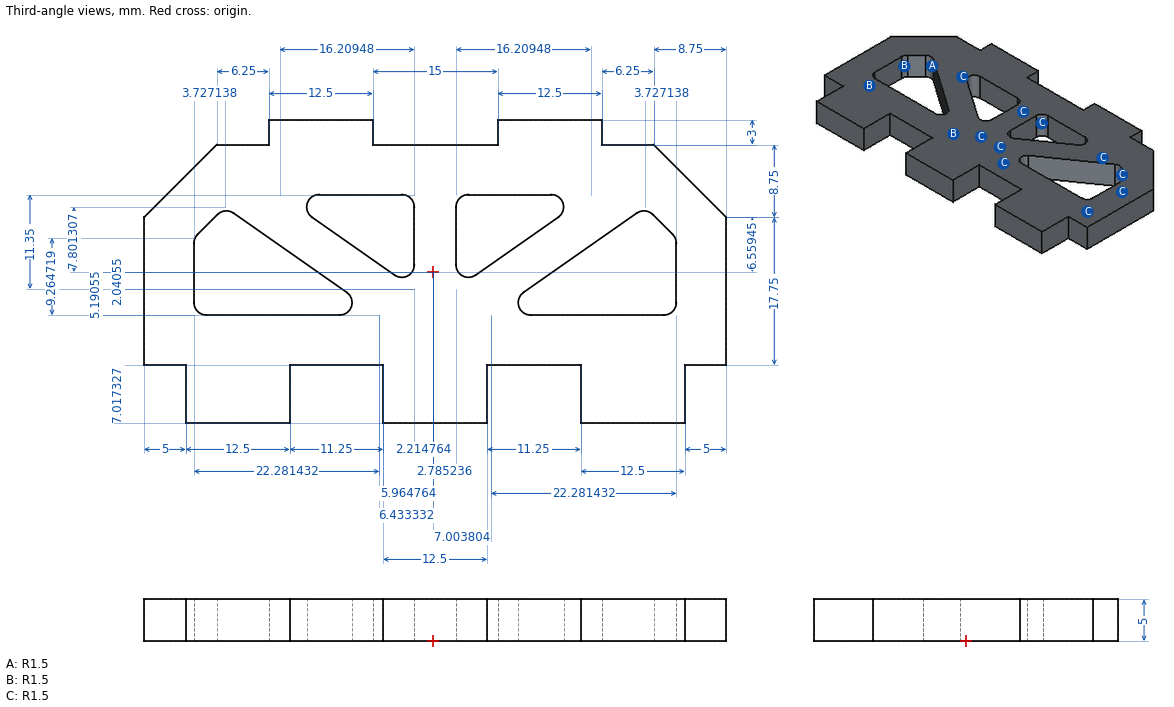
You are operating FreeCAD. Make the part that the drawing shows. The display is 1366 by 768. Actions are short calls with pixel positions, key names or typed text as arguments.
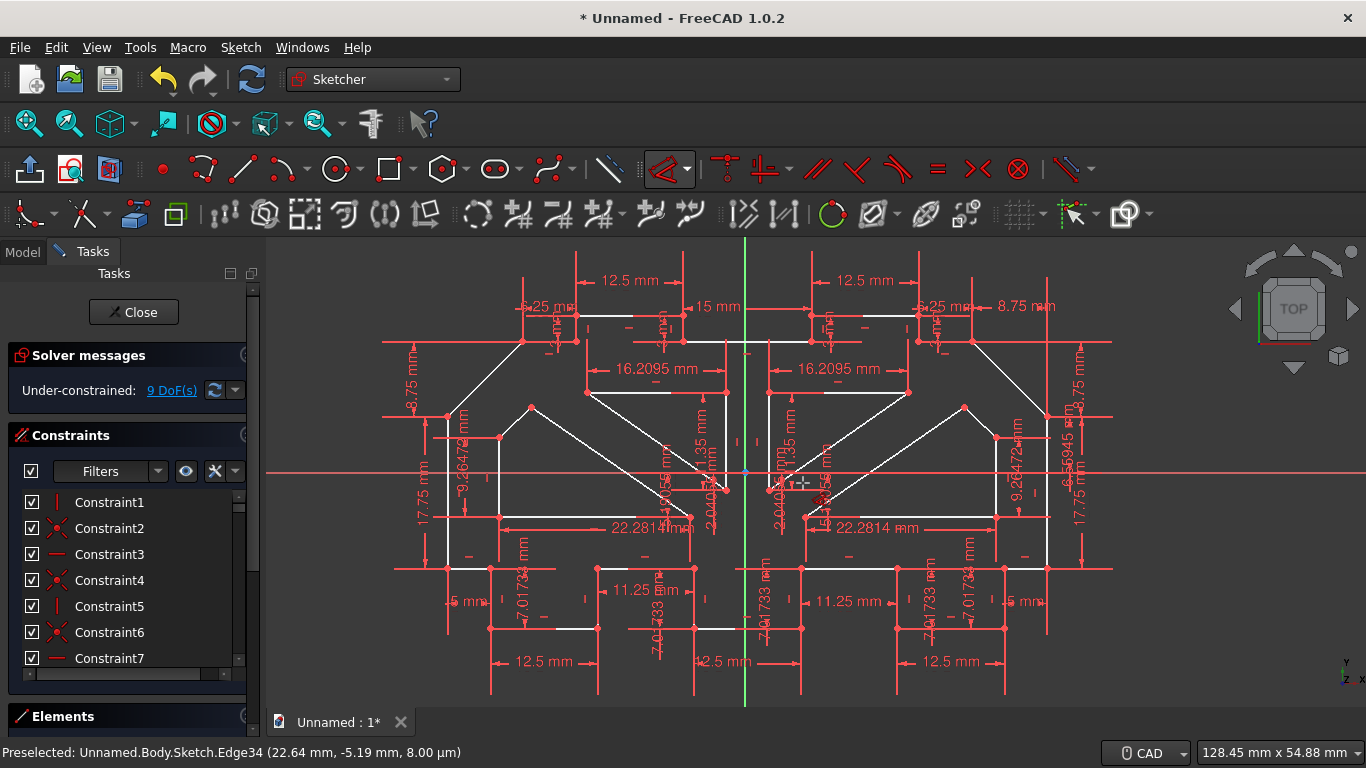
click(694, 569)
click(708, 415)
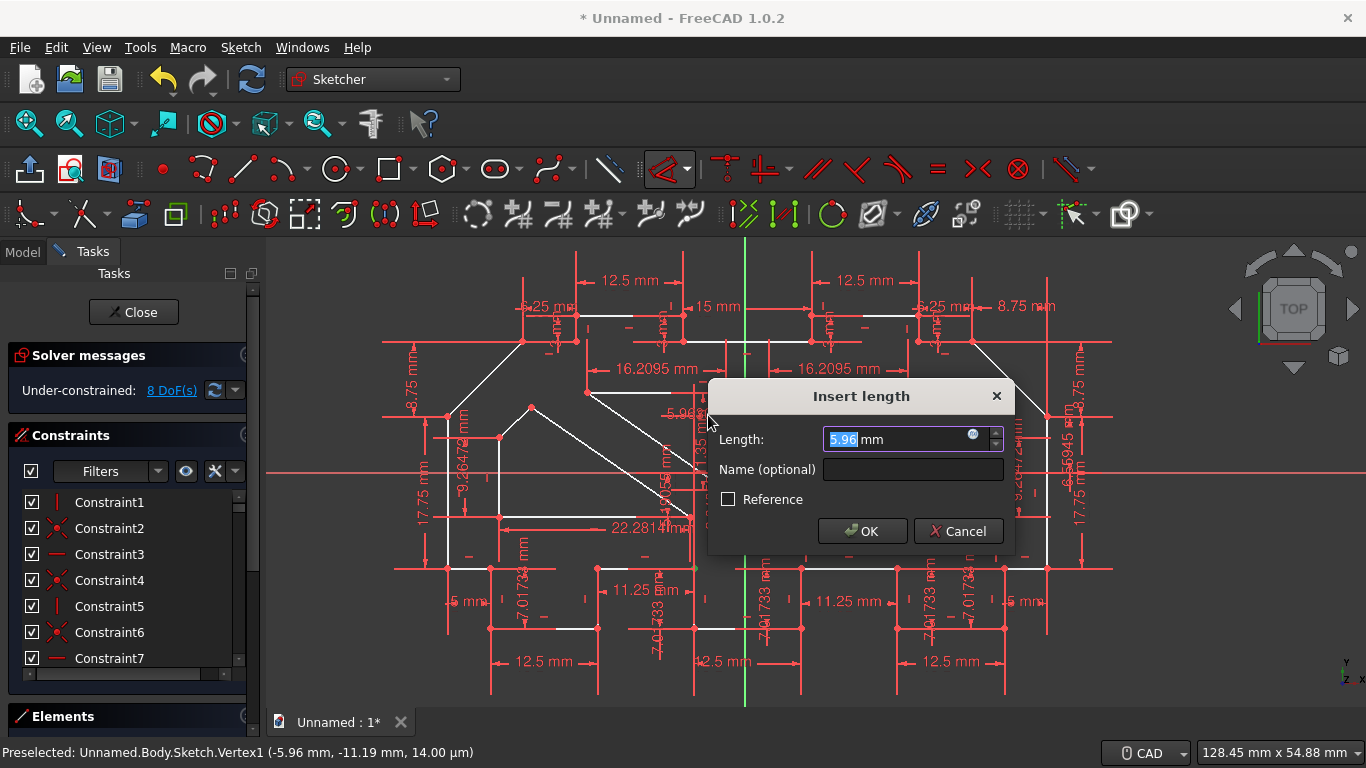
text(5.964764)
key(Return)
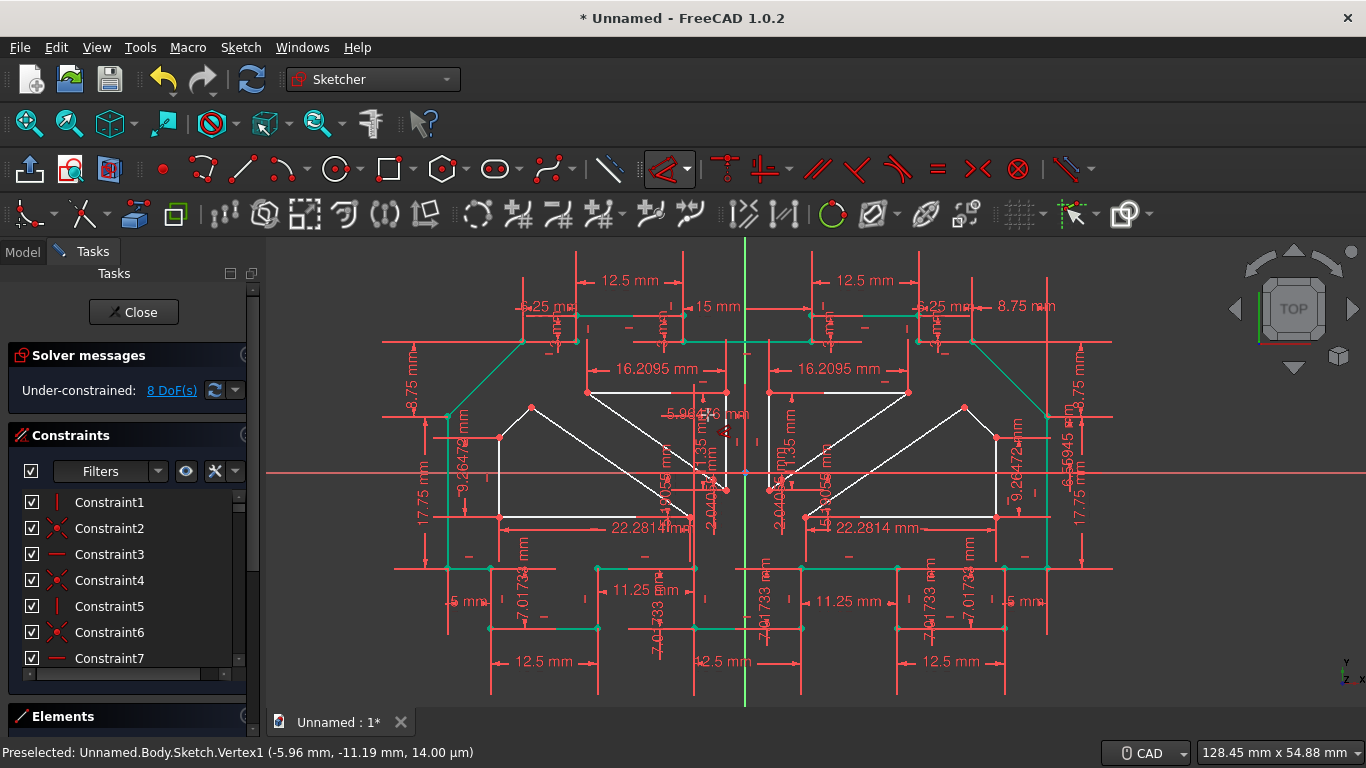
click(690, 517)
click(718, 551)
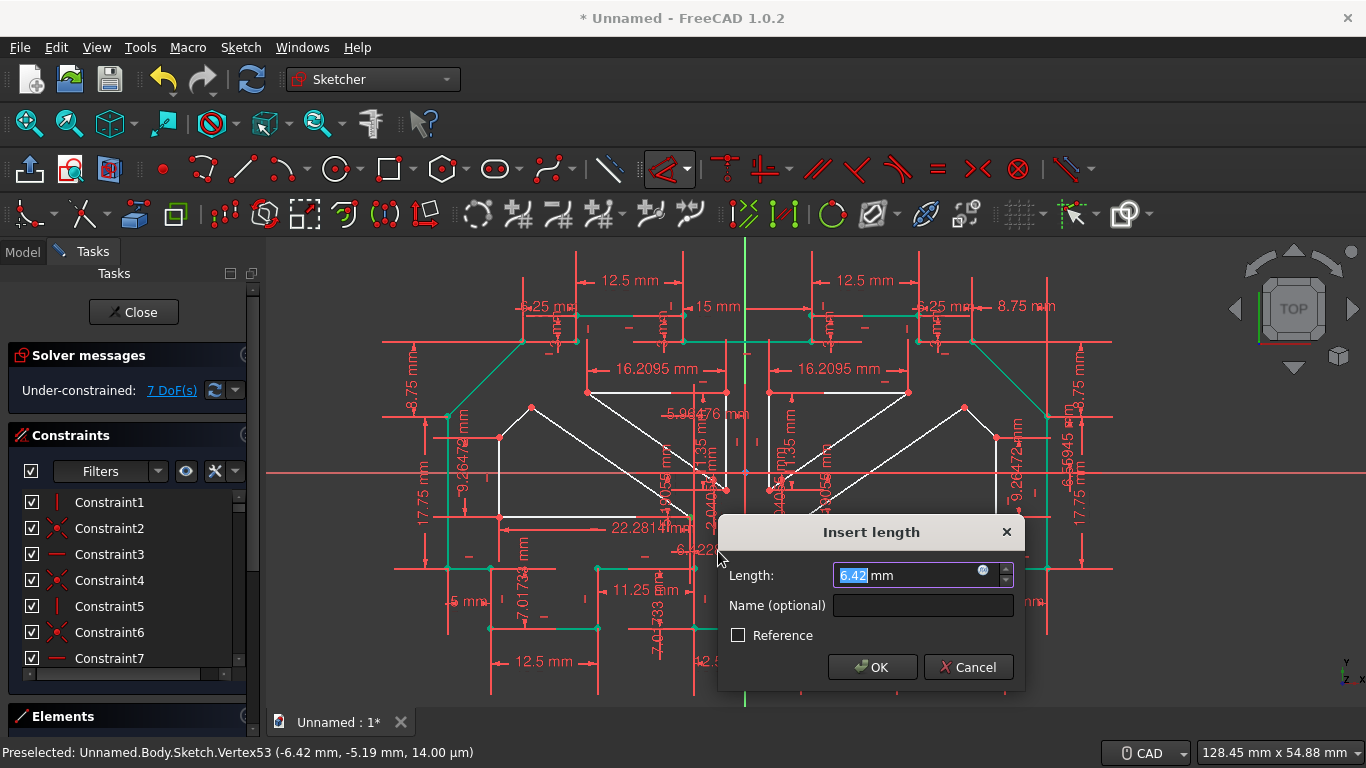
text(6.433332)
key(Return)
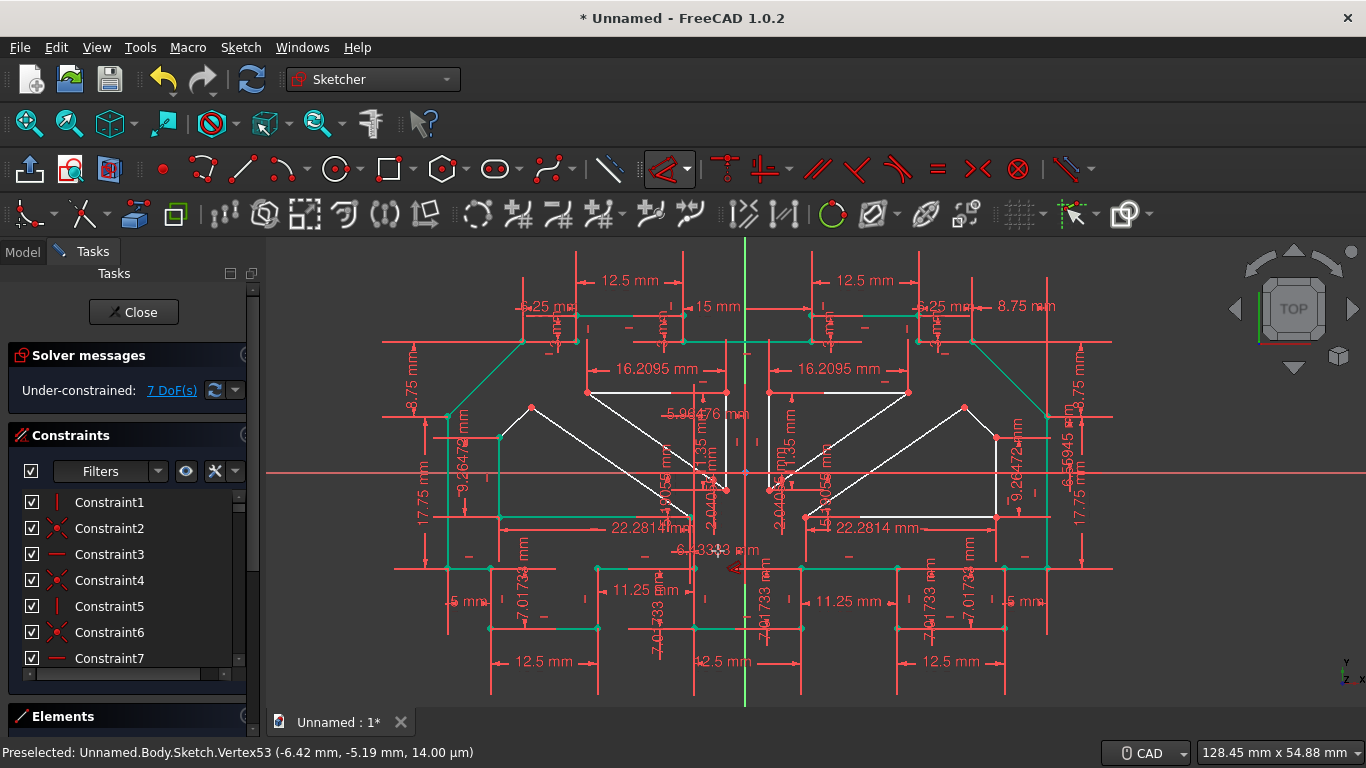
click(531, 407)
click(497, 417)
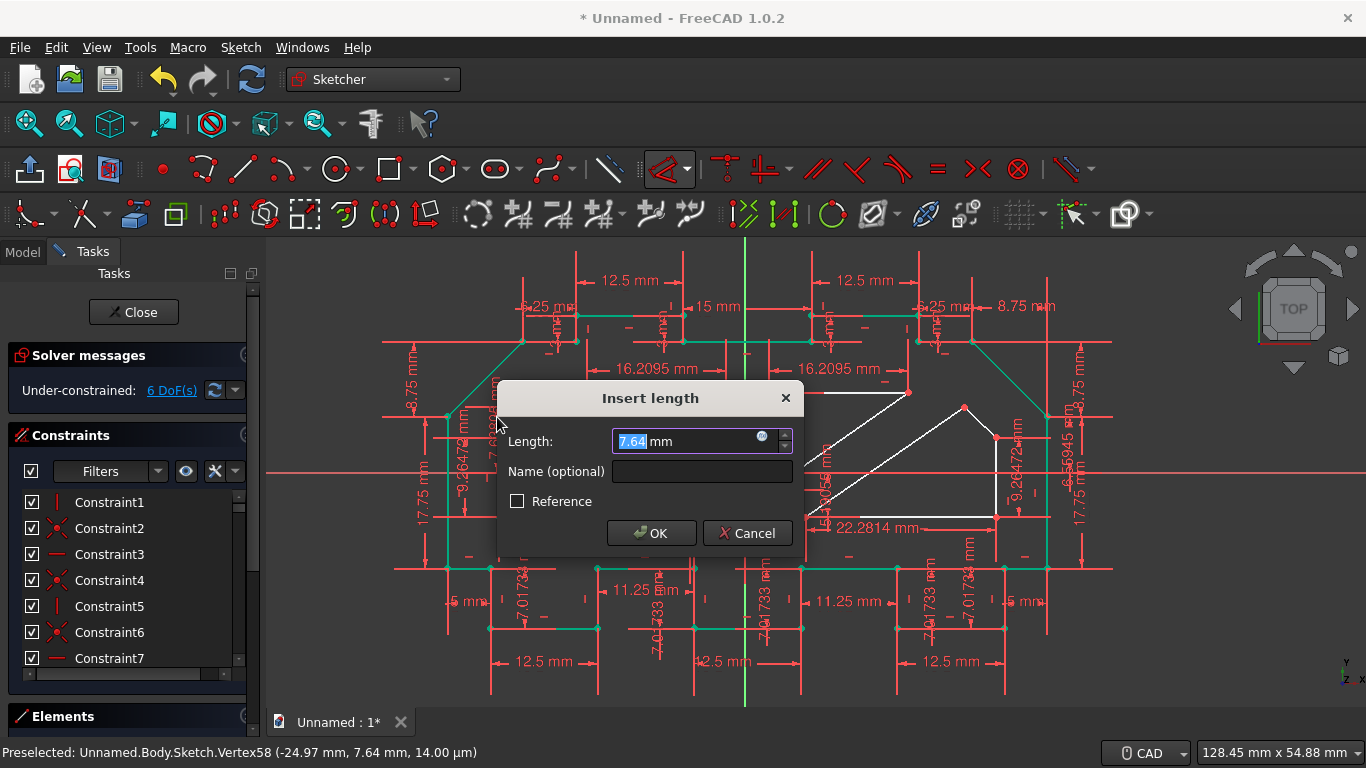
text(7.801307)
key(Return)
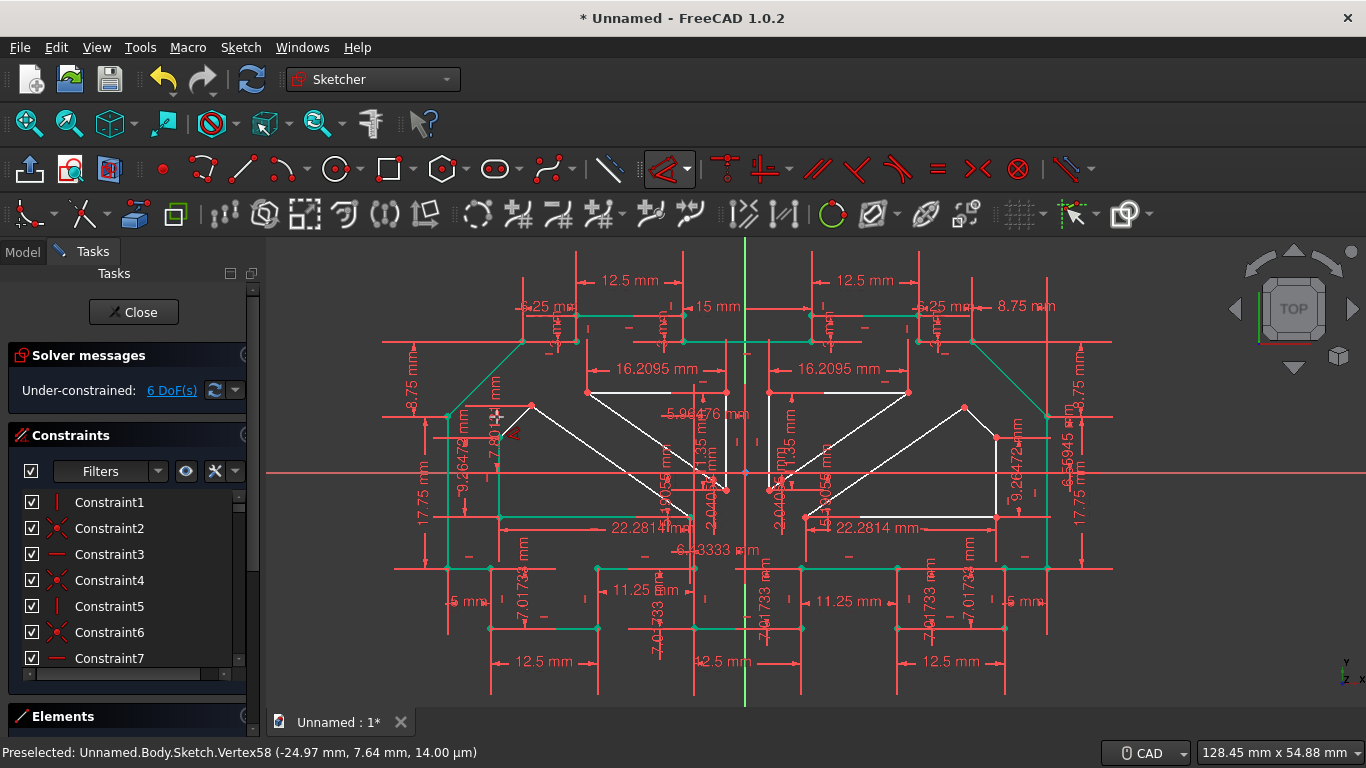
click(806, 517)
click(789, 551)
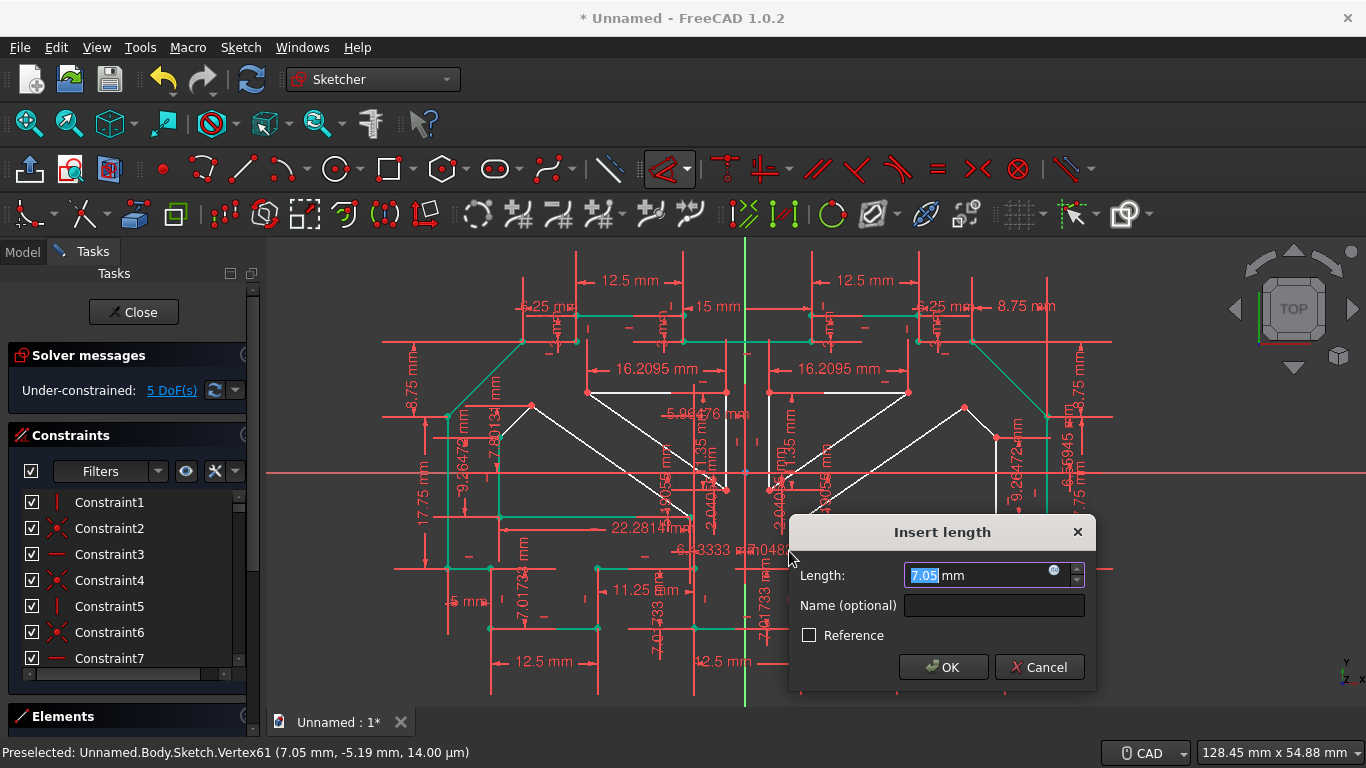
text(7.003804)
key(Return)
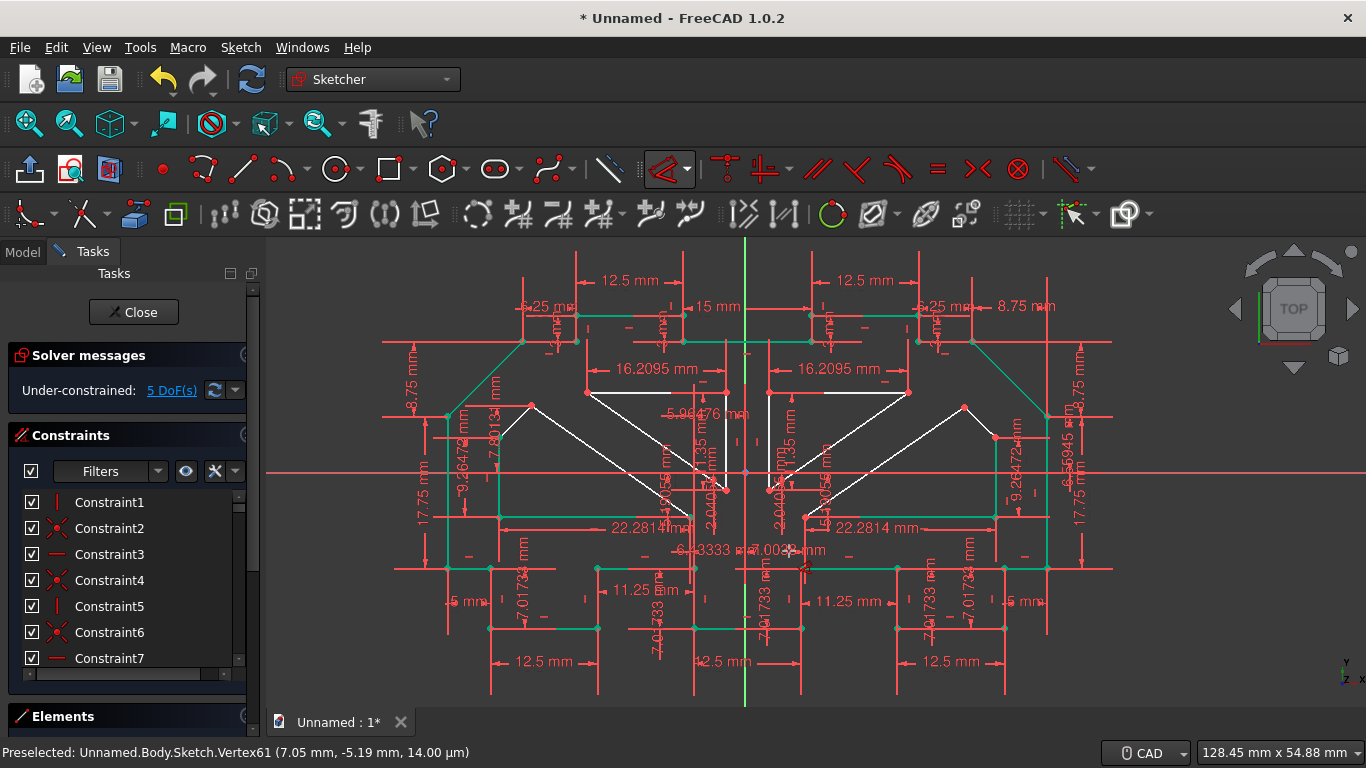
click(964, 407)
click(998, 417)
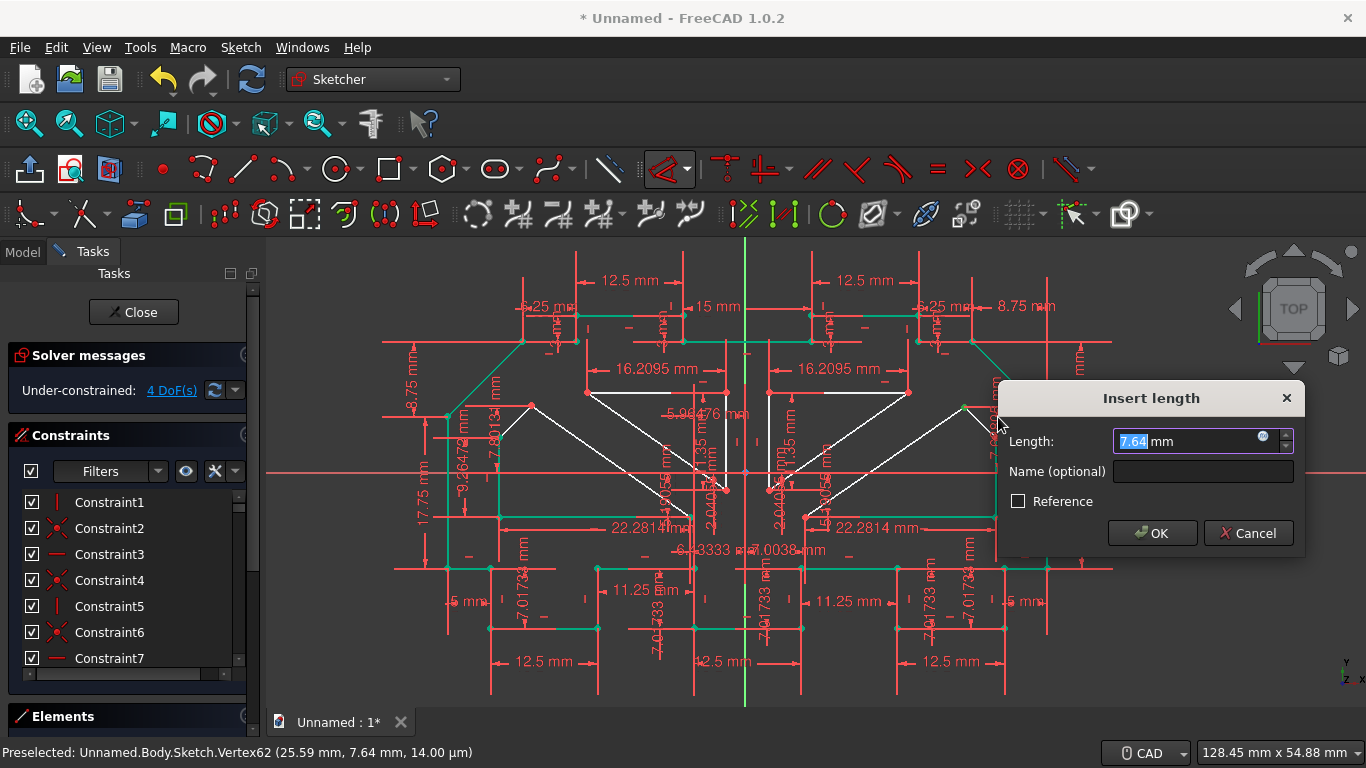
text(7.801307)
key(Return)